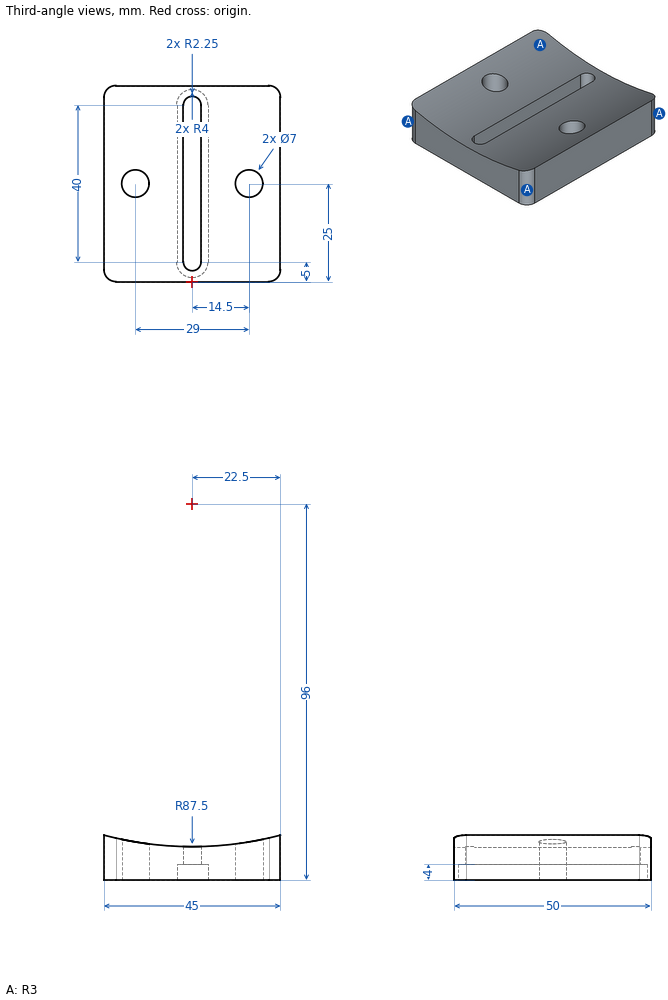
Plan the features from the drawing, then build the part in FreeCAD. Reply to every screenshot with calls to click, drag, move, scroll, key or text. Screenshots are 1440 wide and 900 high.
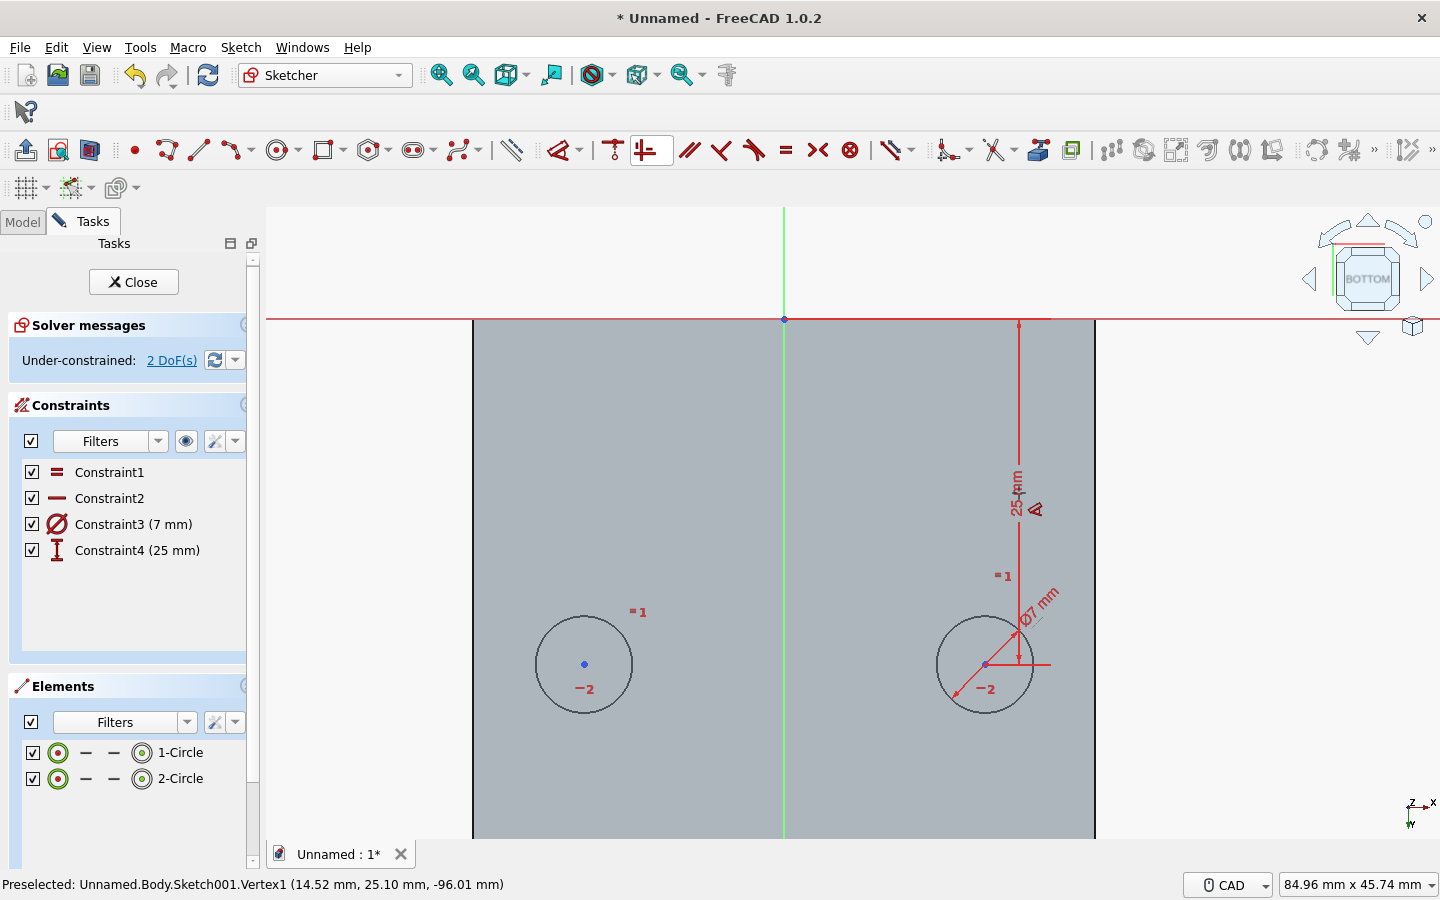
click(985, 665)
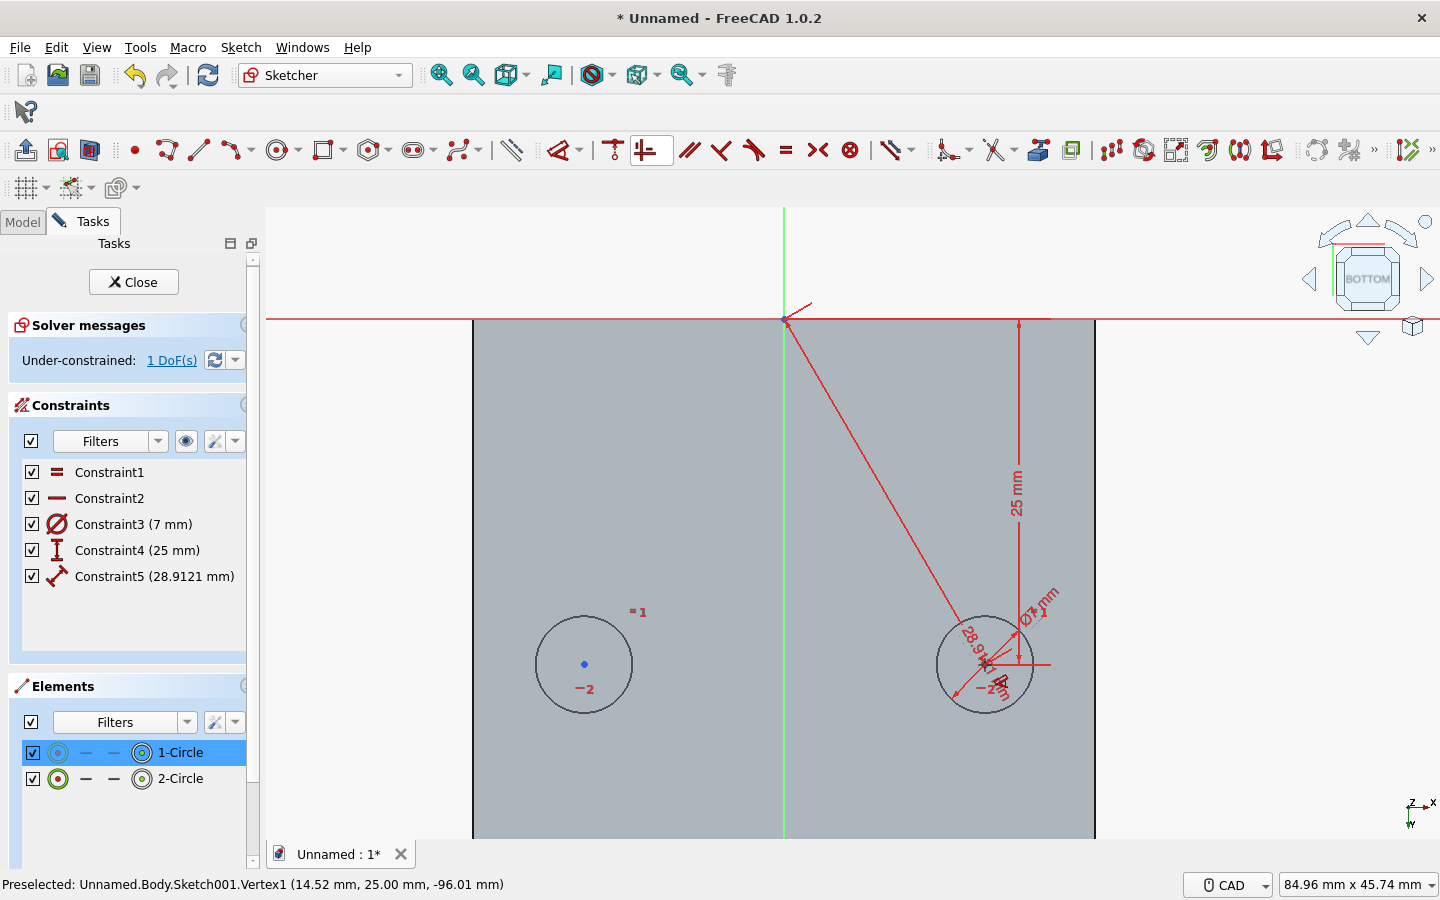
click(584, 665)
click(692, 699)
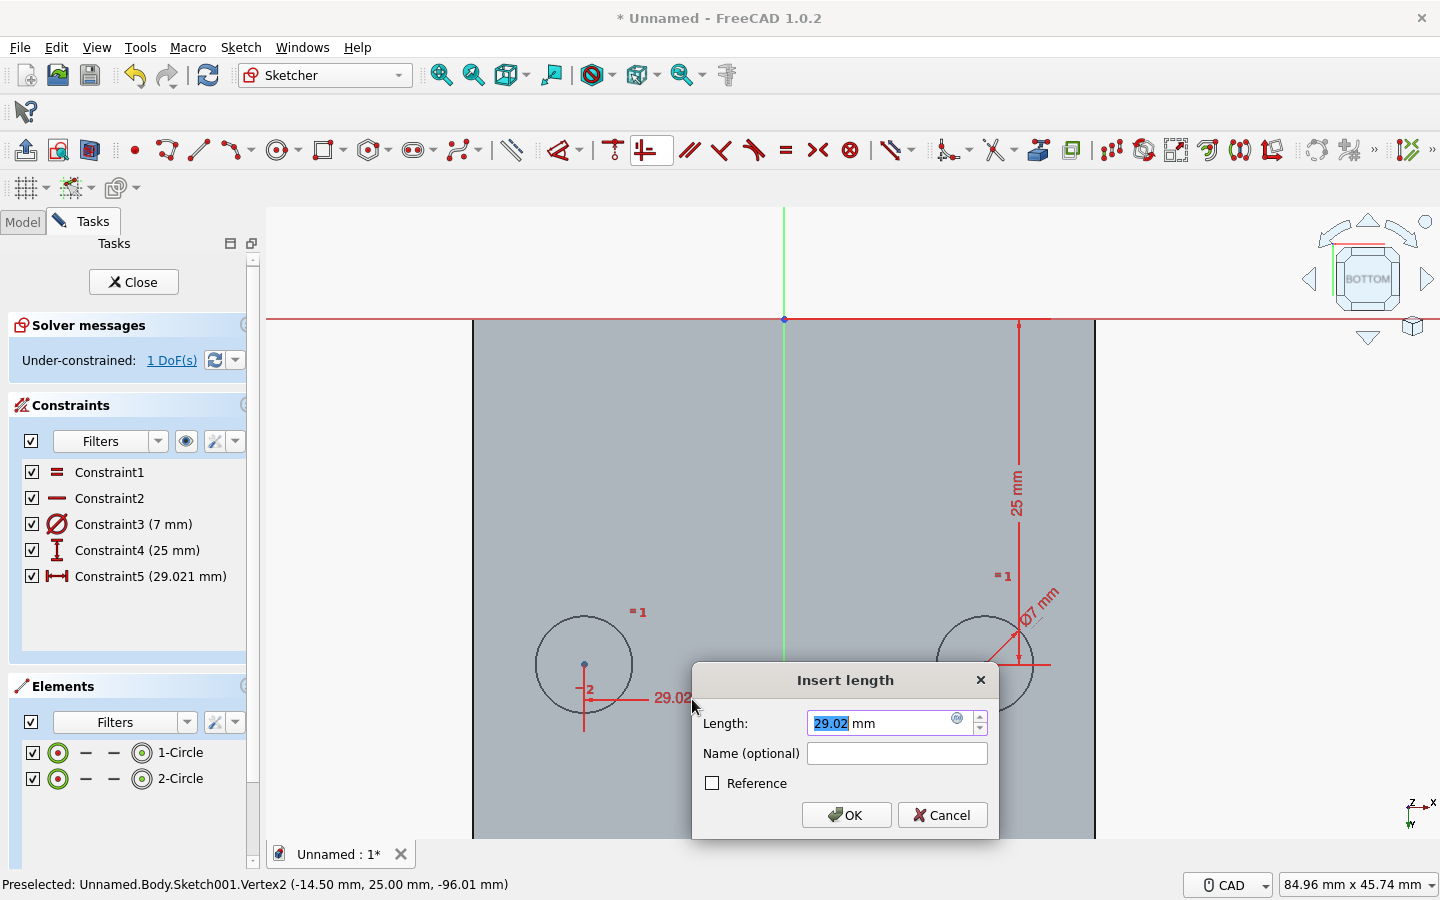
text(29)
key(Return)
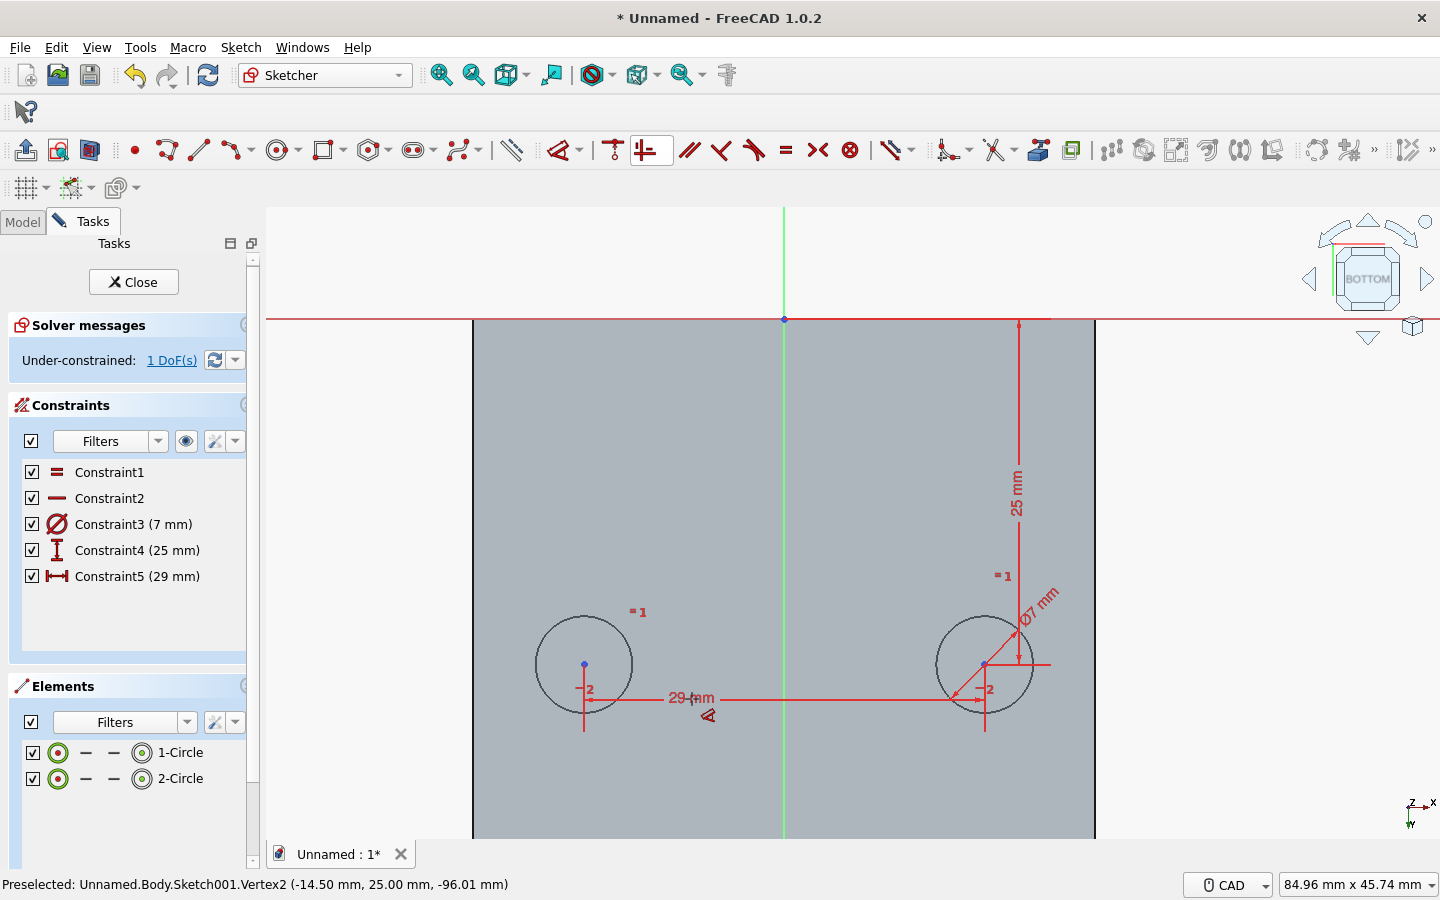
click(985, 665)
click(885, 285)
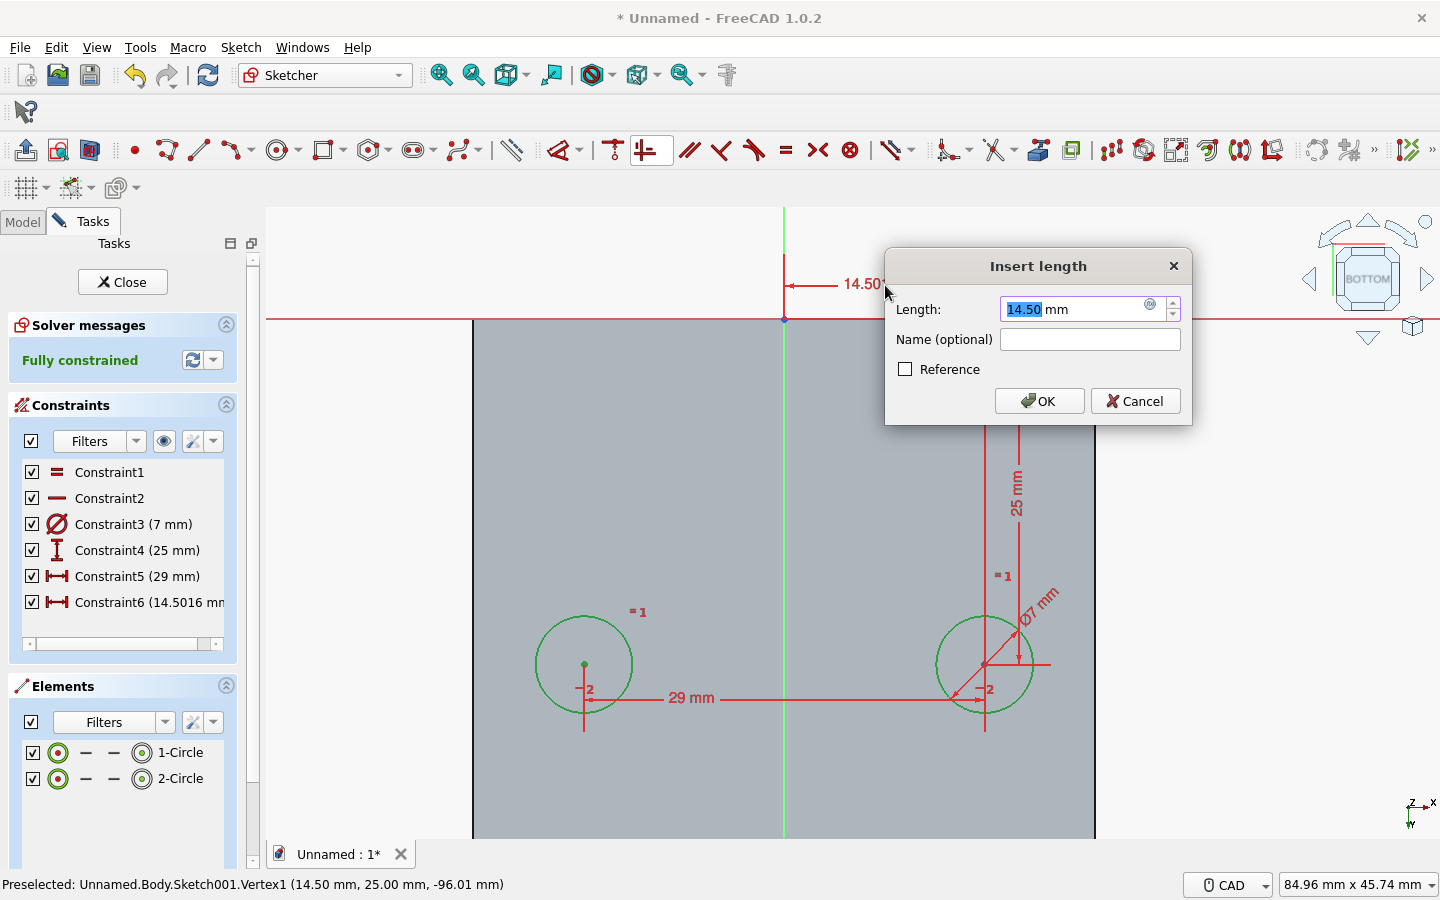
text(14.5)
key(Return)
key(Escape)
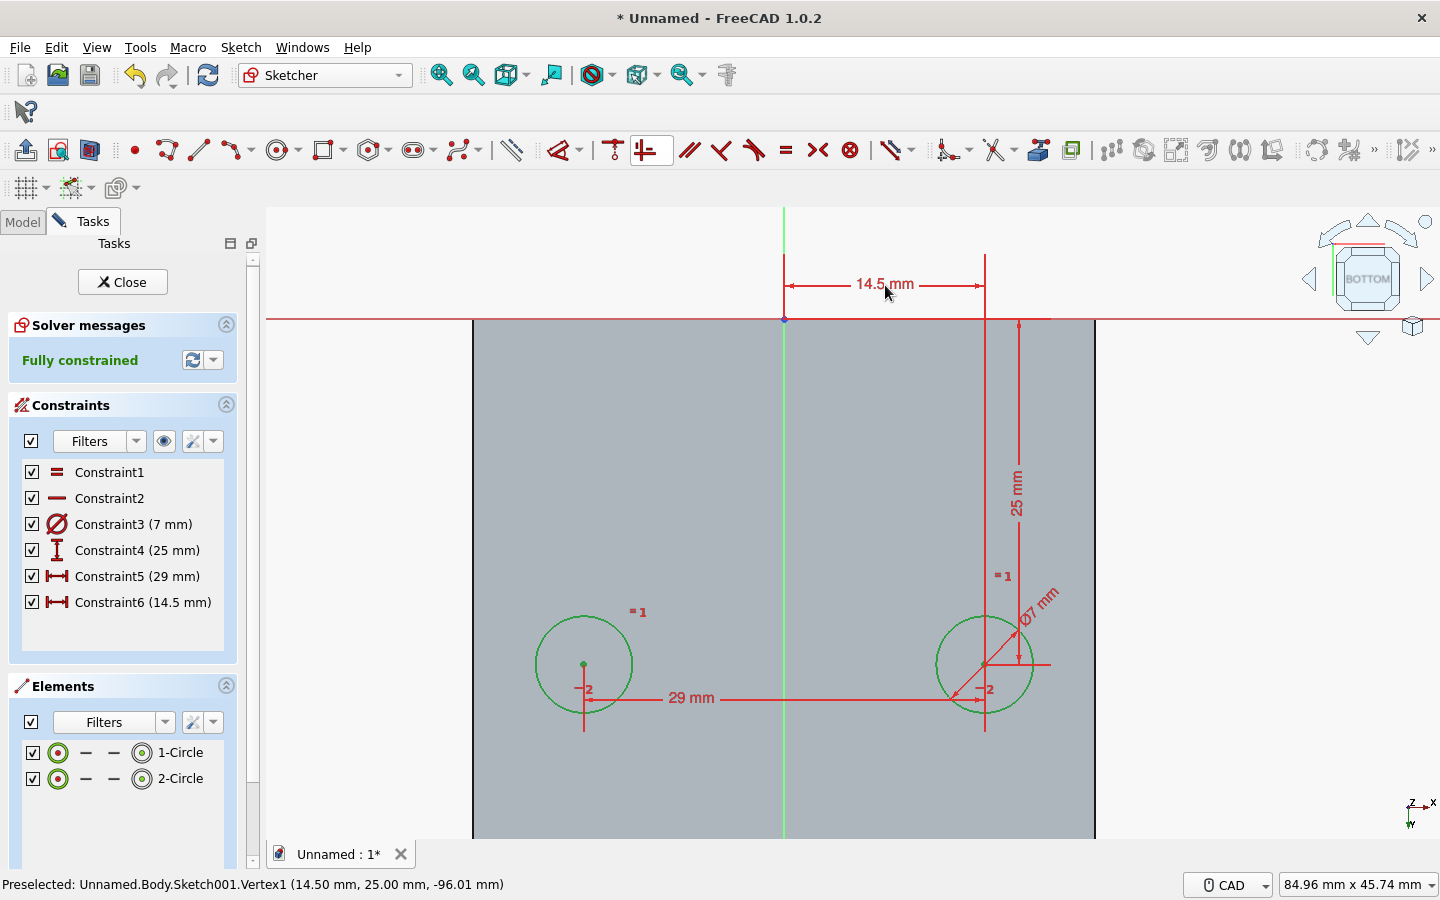
click(123, 282)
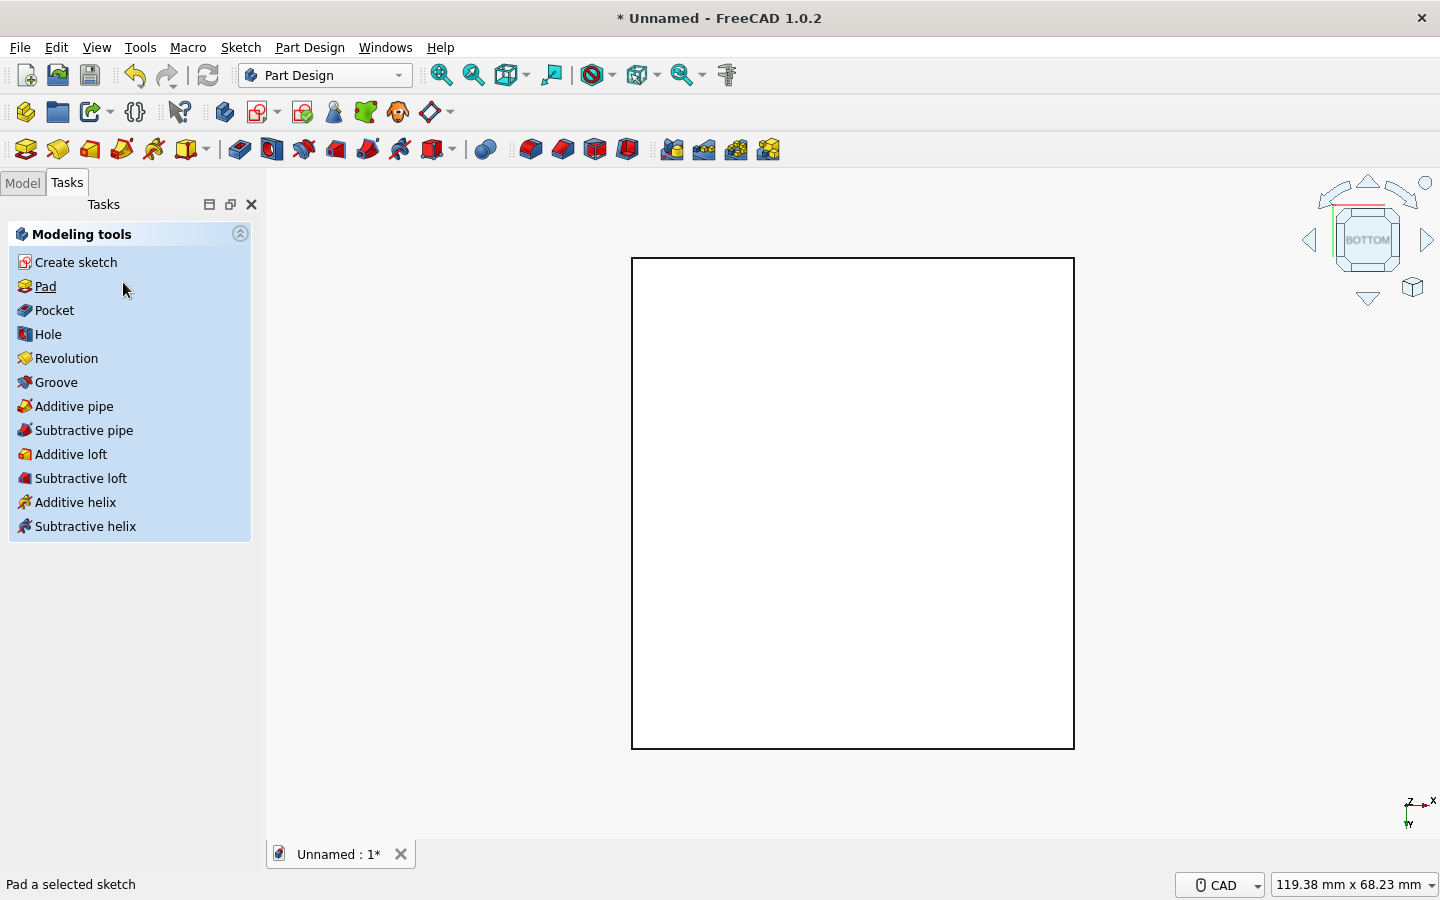
click(240, 150)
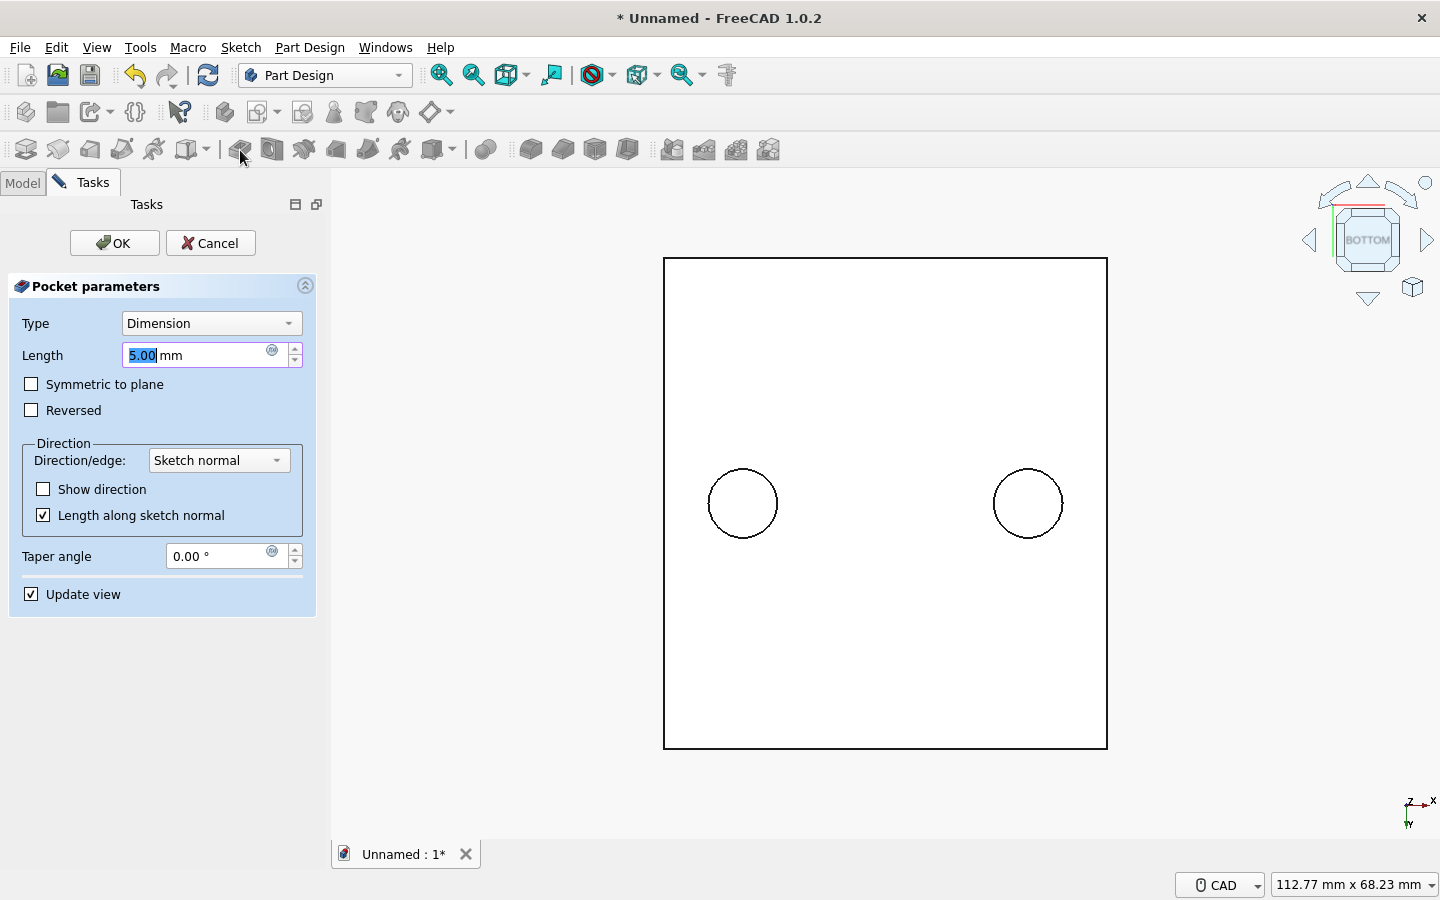
click(212, 324)